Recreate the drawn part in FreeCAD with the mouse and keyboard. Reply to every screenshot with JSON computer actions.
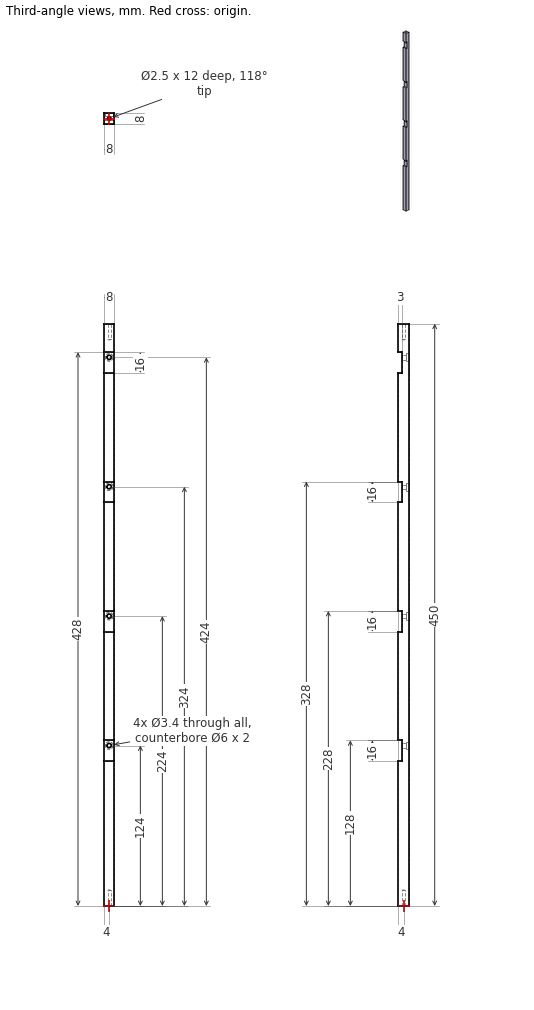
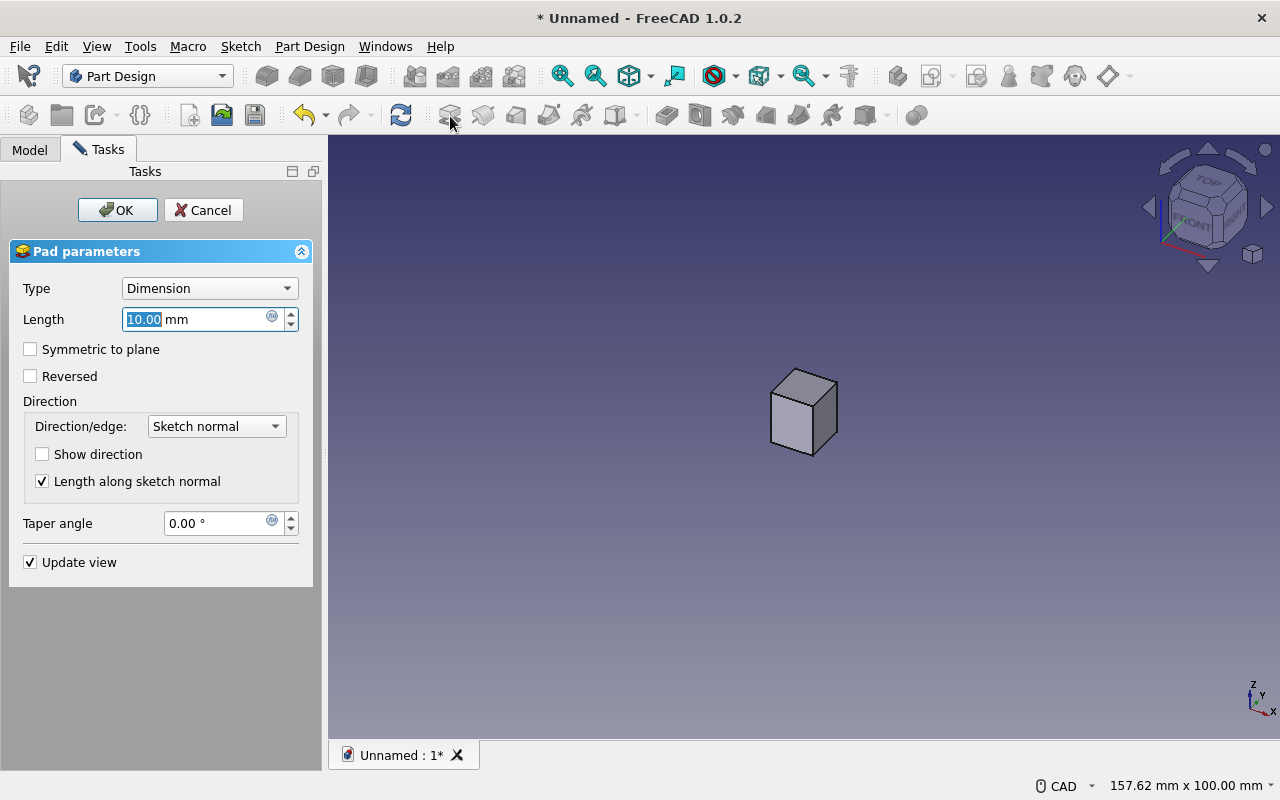
{"action": "type", "text": "450"}
{"action": "key", "text": "Tab"}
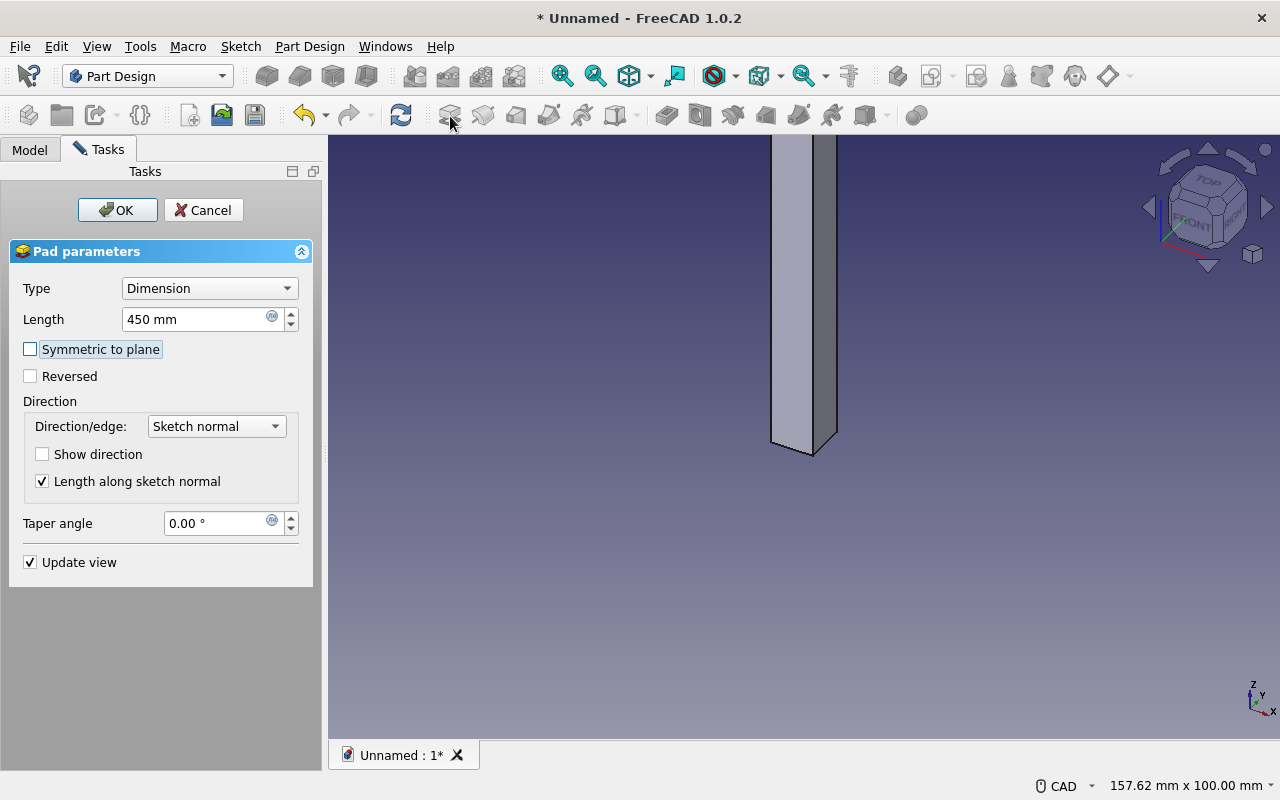
{"action": "left_click", "coordinate": [118, 210]}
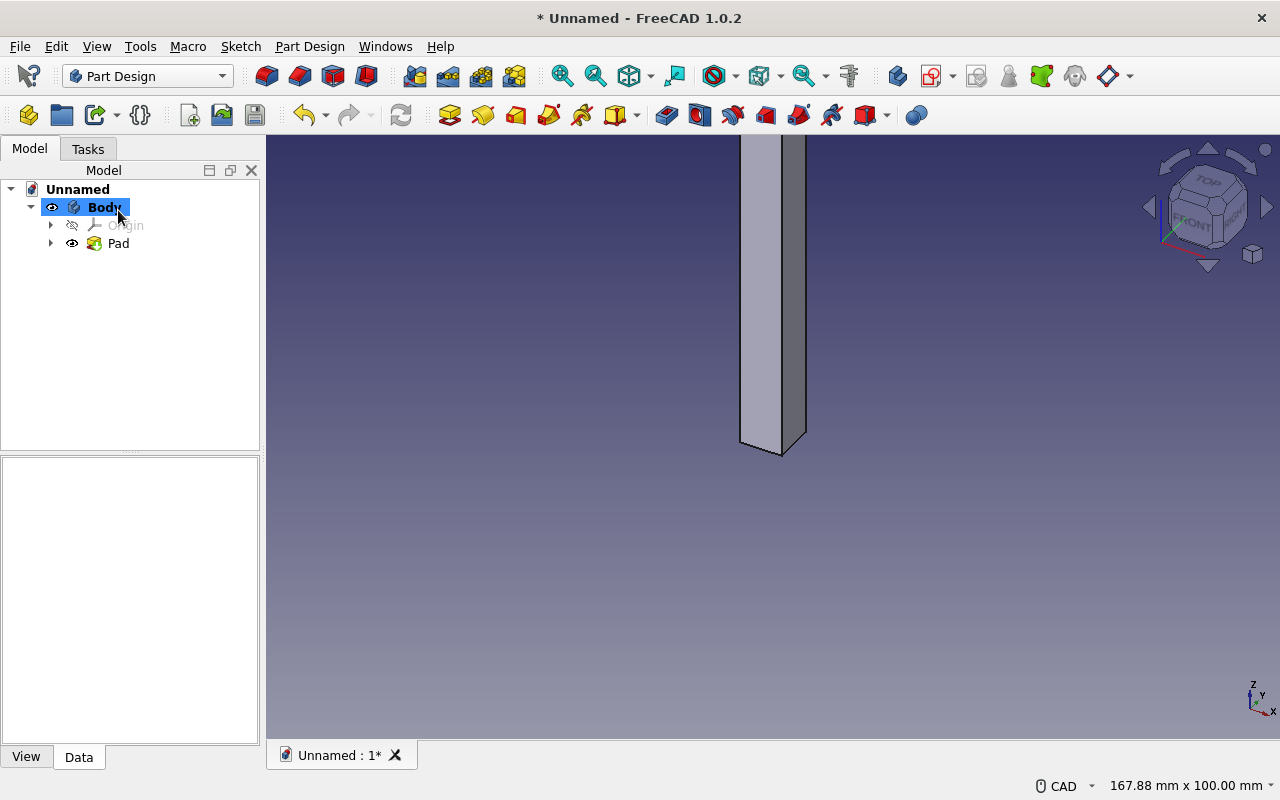
{"action": "key", "text": "v f"}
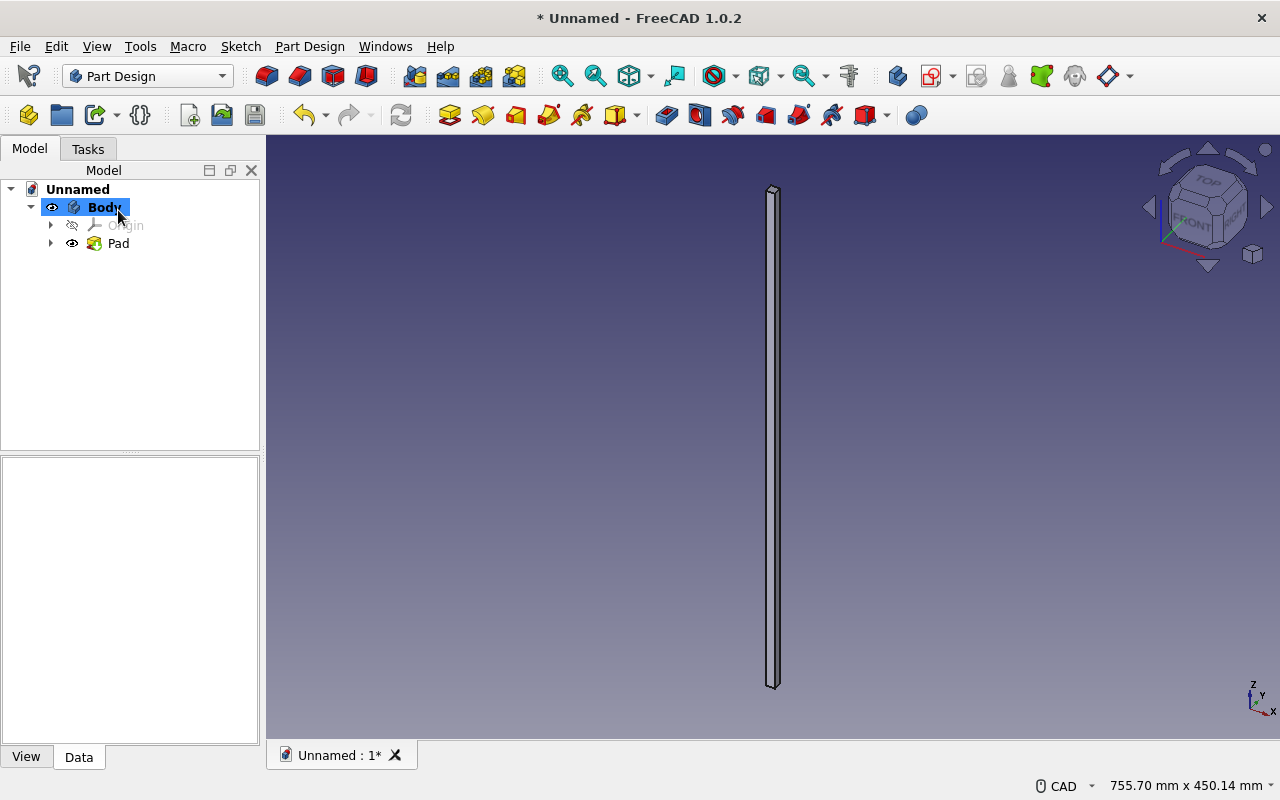
{"action": "scroll", "coordinate": [770, 227], "scroll_direction": "up", "scroll_amount": 5}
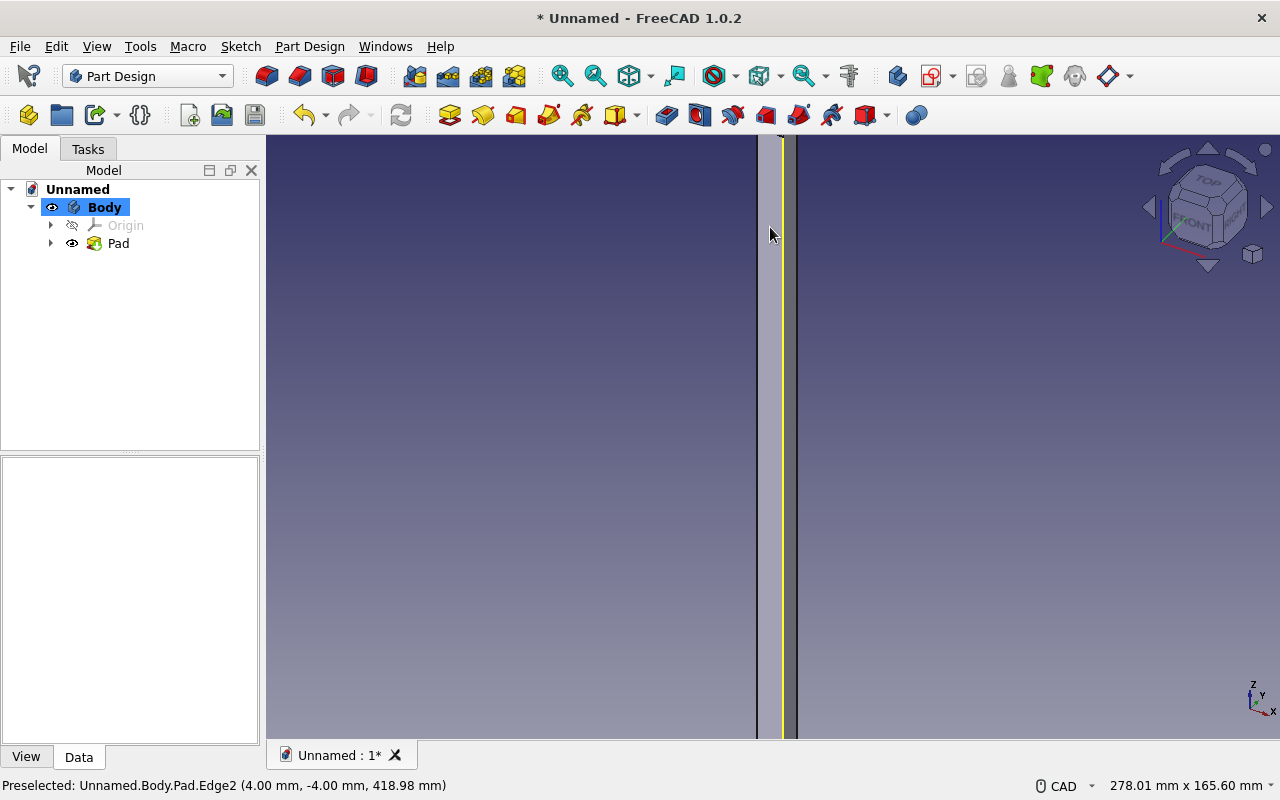
{"action": "left_click", "coordinate": [770, 228]}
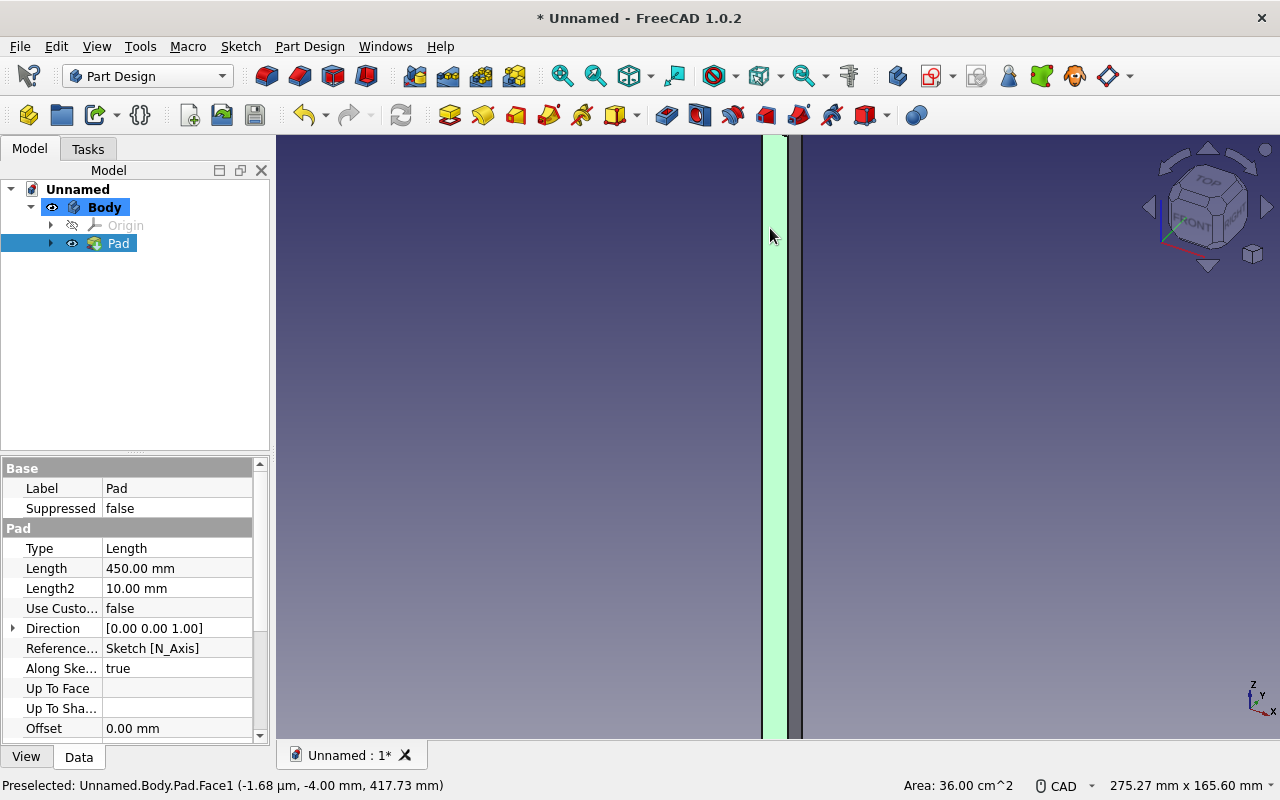
{"action": "left_click", "coordinate": [930, 76]}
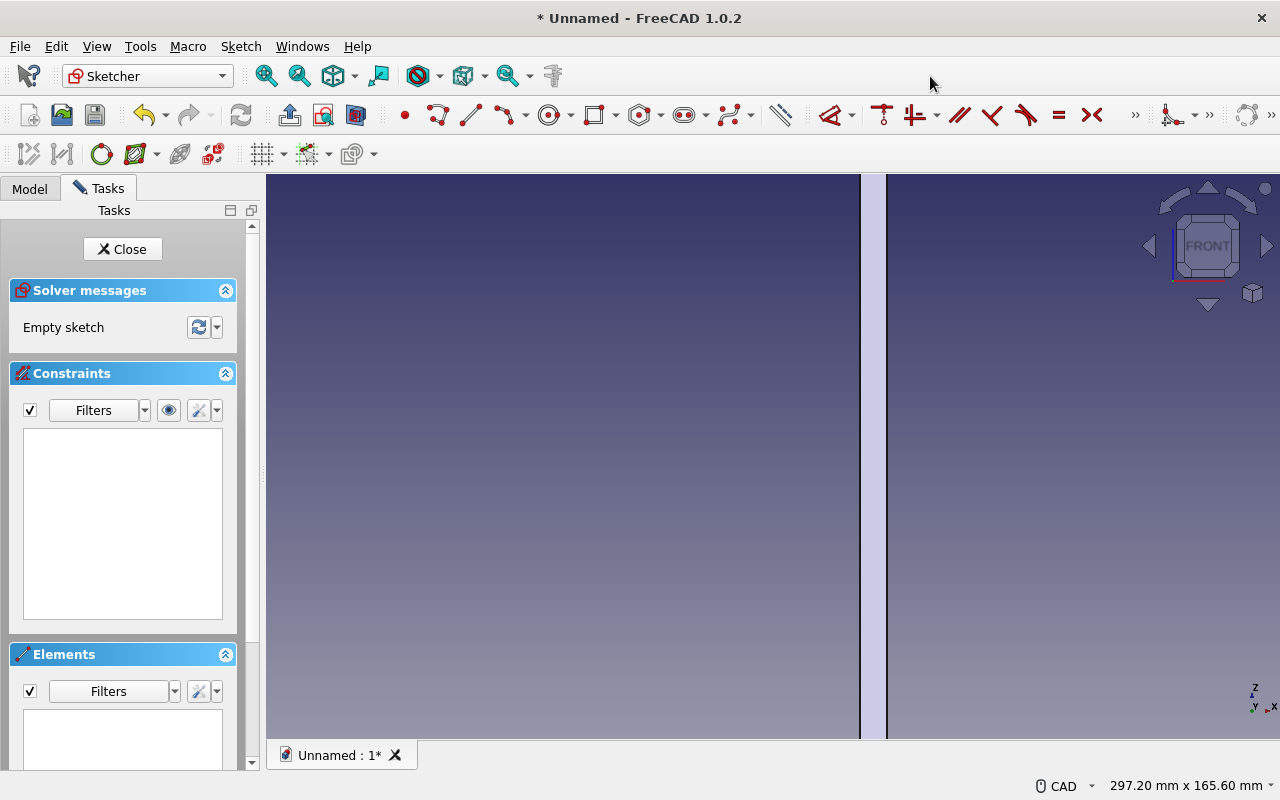
{"action": "scroll", "coordinate": [704, 456], "scroll_direction": "down", "scroll_amount": 5}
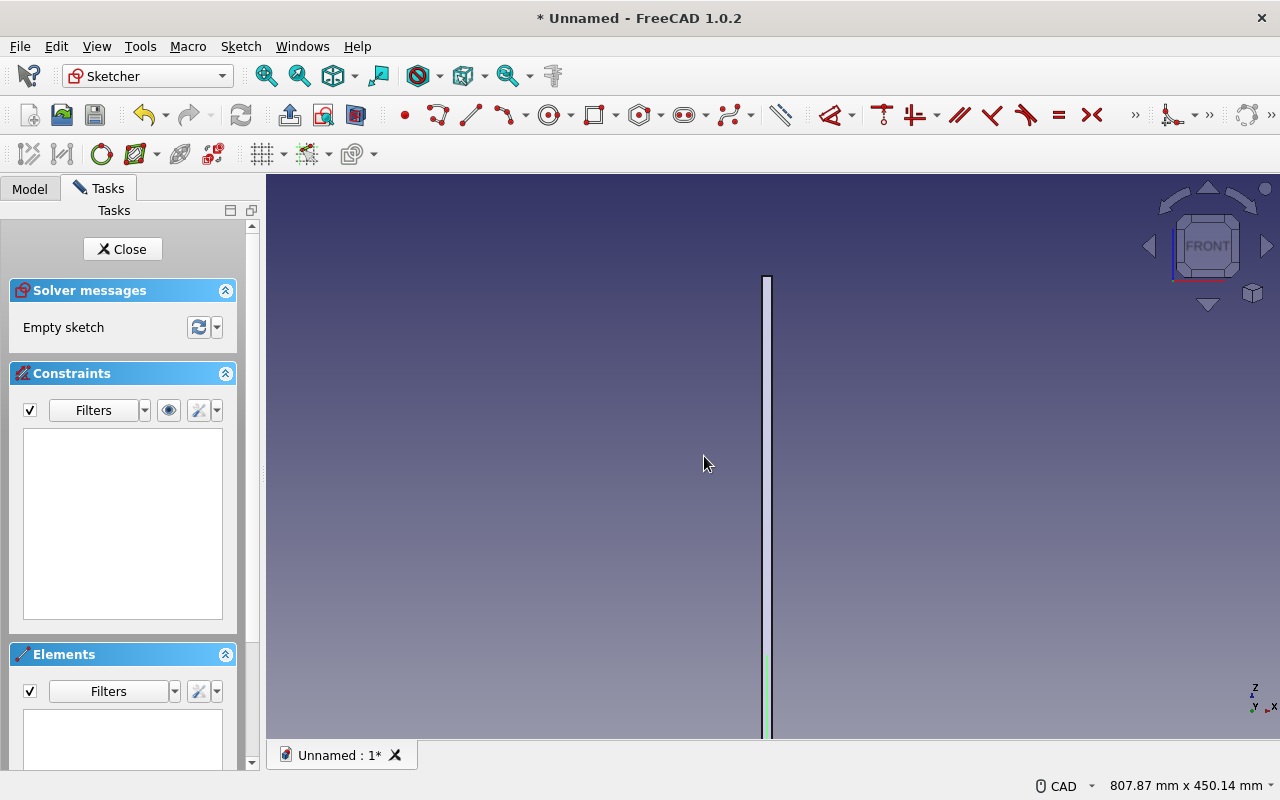
{"action": "scroll", "coordinate": [771, 304], "scroll_direction": "up", "scroll_amount": 14}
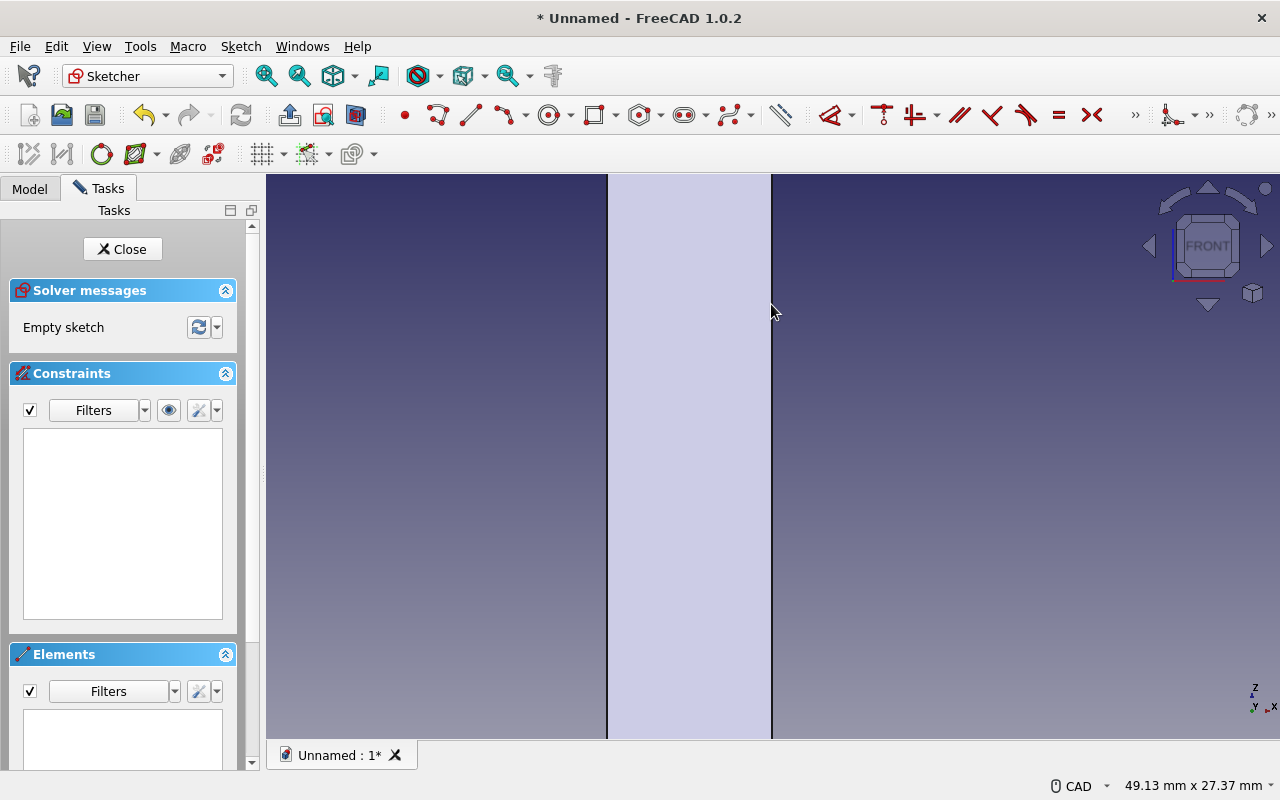
{"action": "key", "text": "g r"}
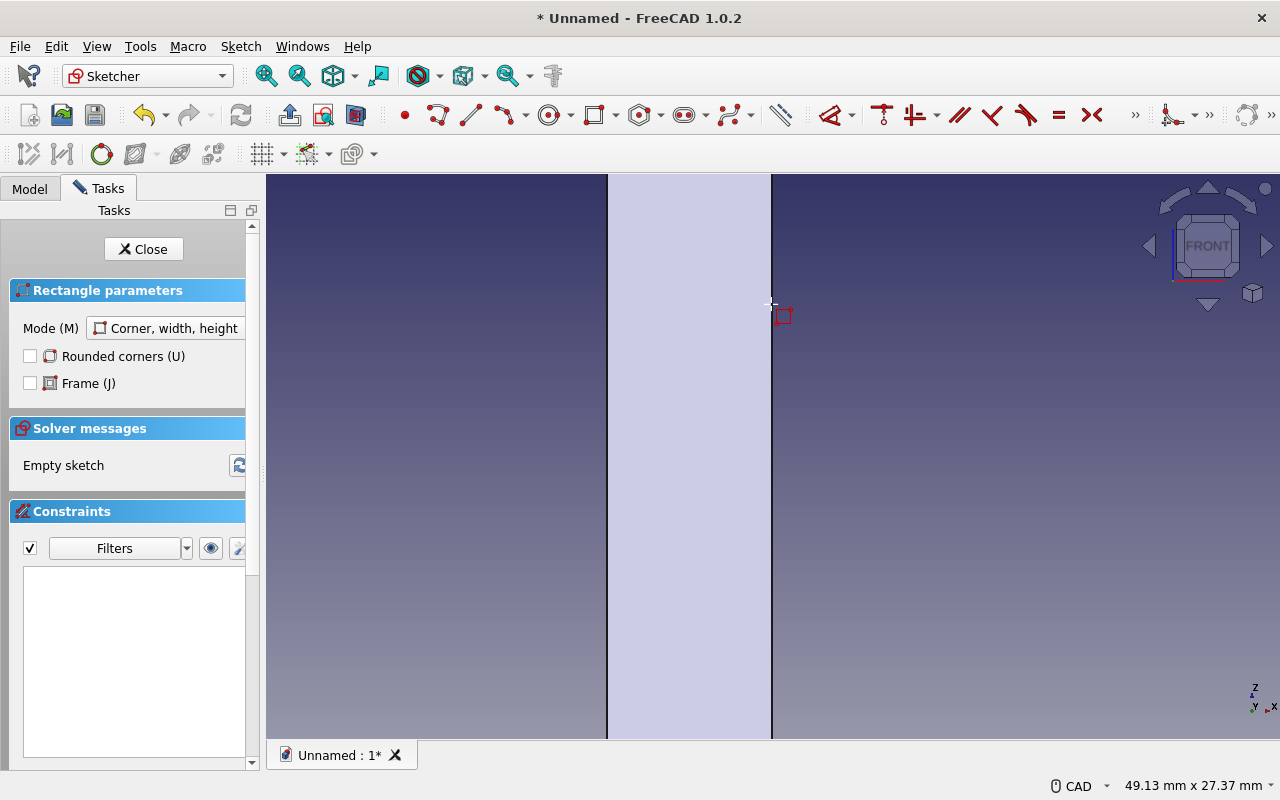
{"action": "left_click", "coordinate": [607, 290]}
{"action": "mouse_move", "coordinate": [772, 620]}